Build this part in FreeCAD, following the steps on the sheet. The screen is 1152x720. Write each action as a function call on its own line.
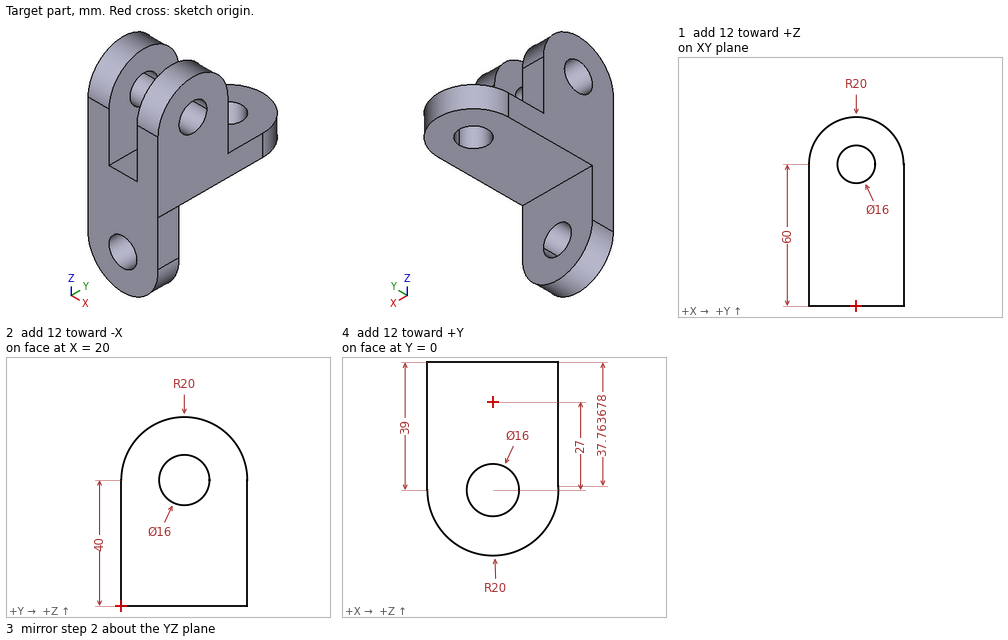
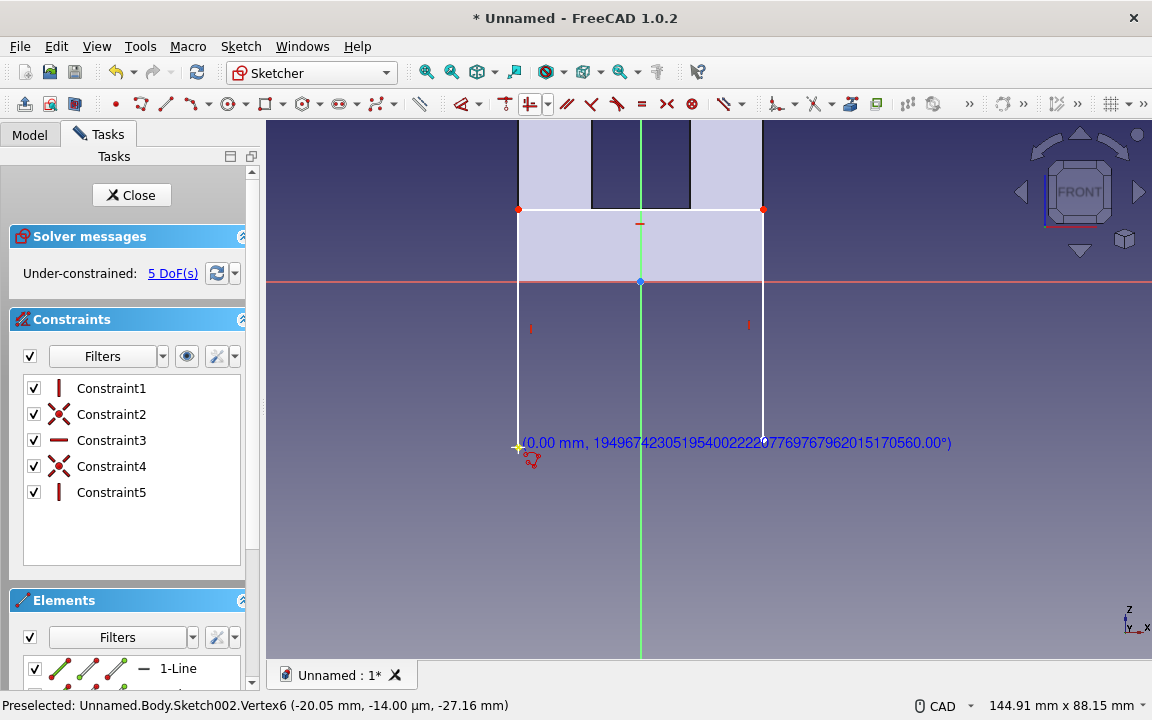
key(g)
key(3)
key(a)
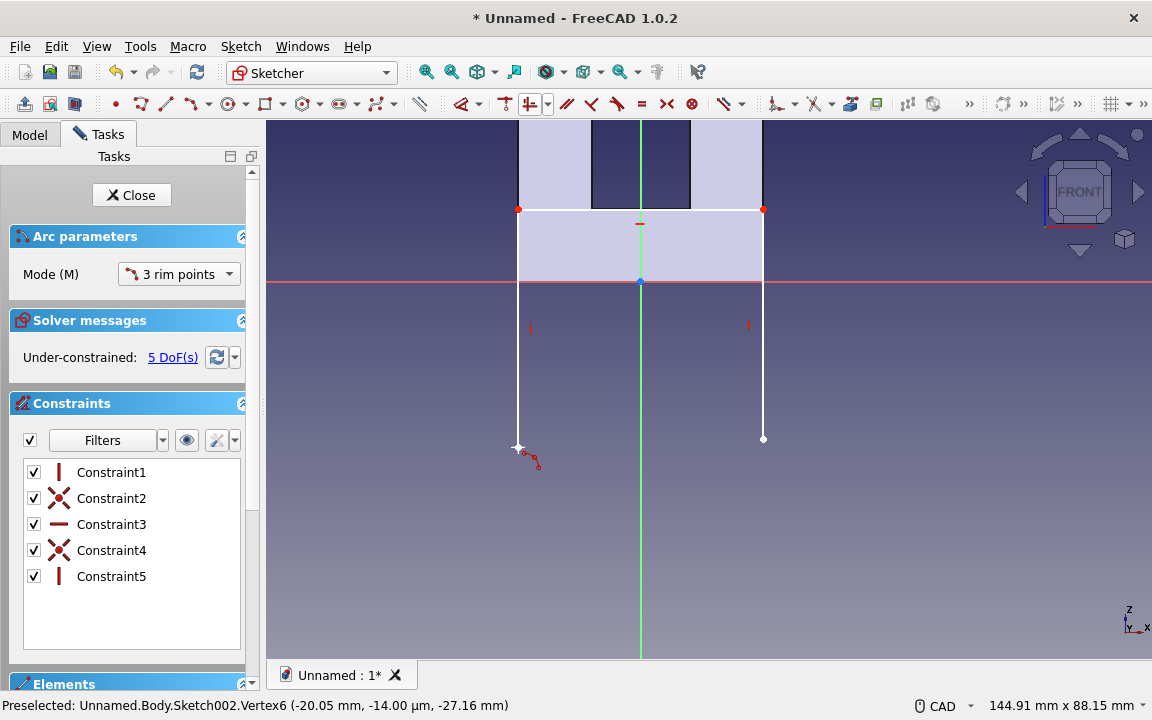
click(518, 448)
click(763, 440)
click(606, 564)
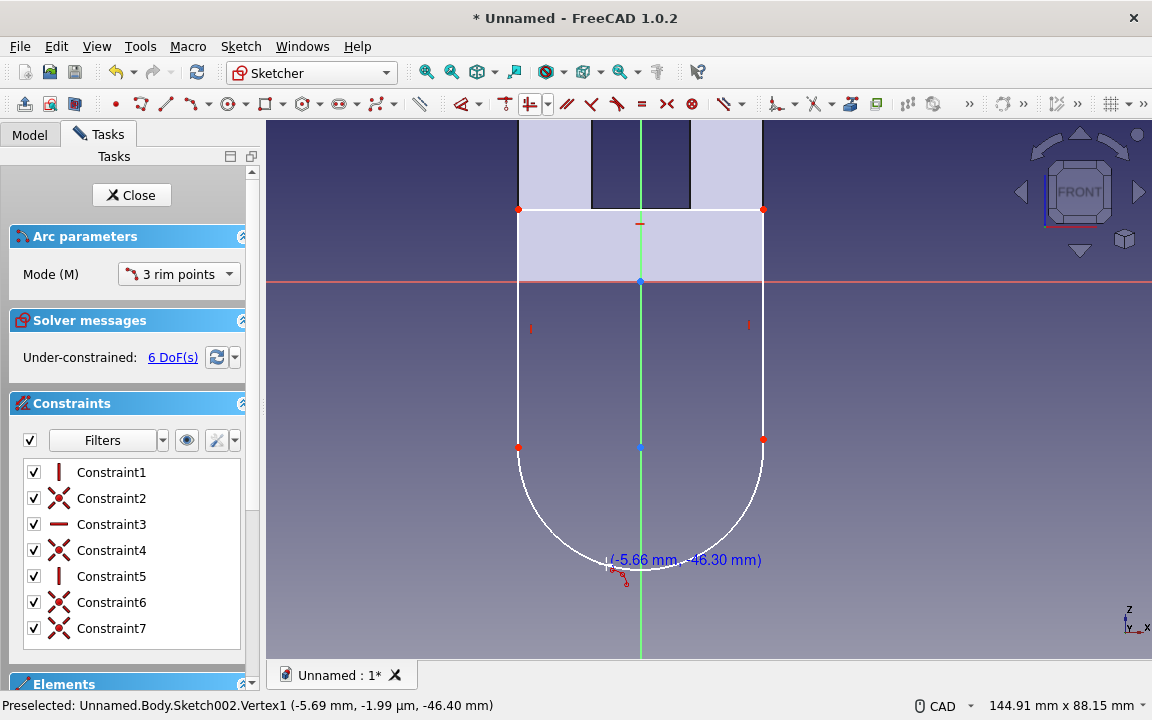
click(228, 104)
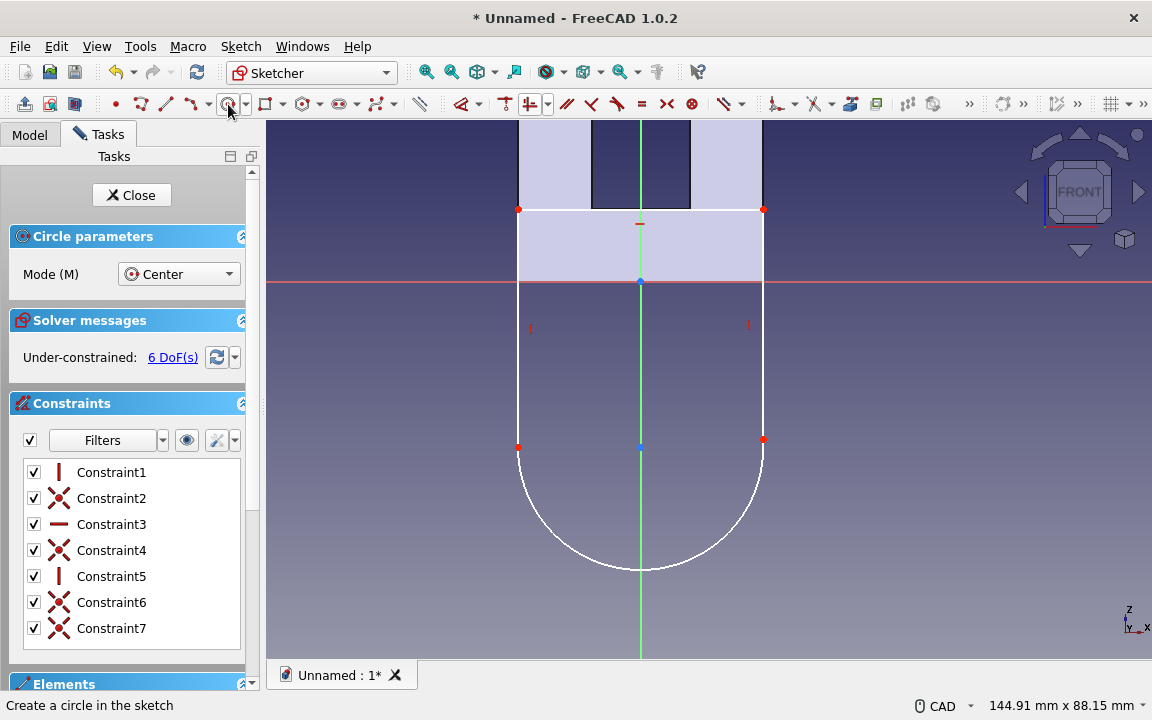
click(641, 447)
move(675, 412)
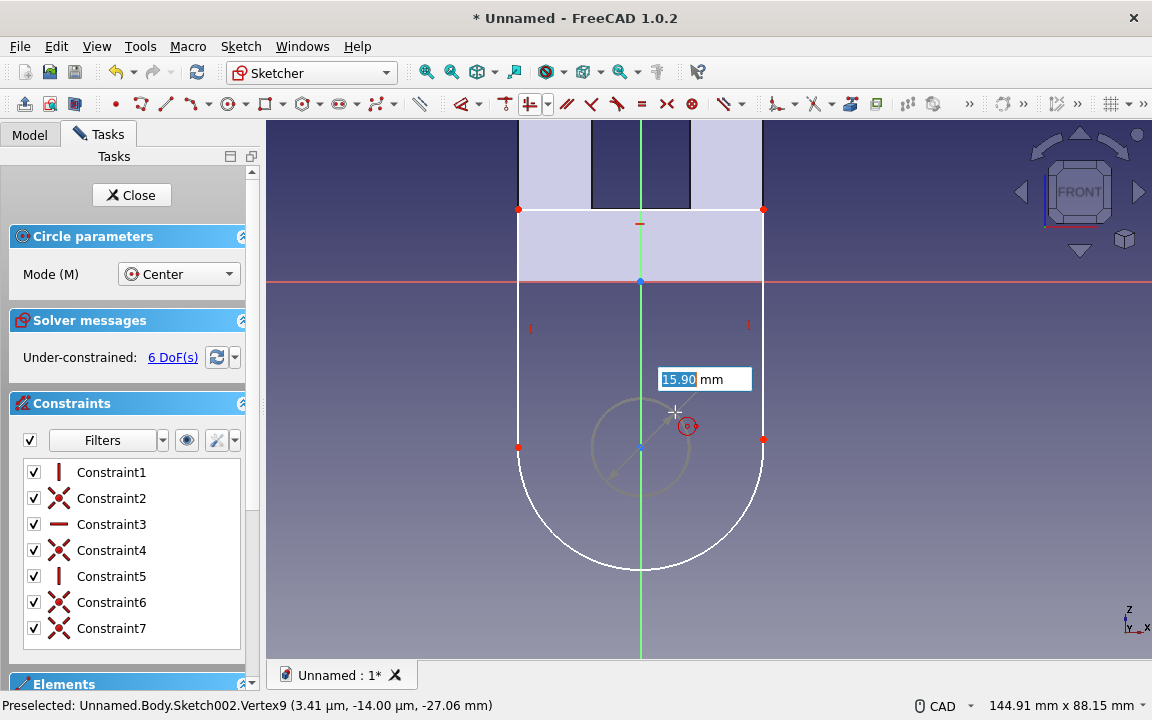
text(16)
key(Return)
key(Escape)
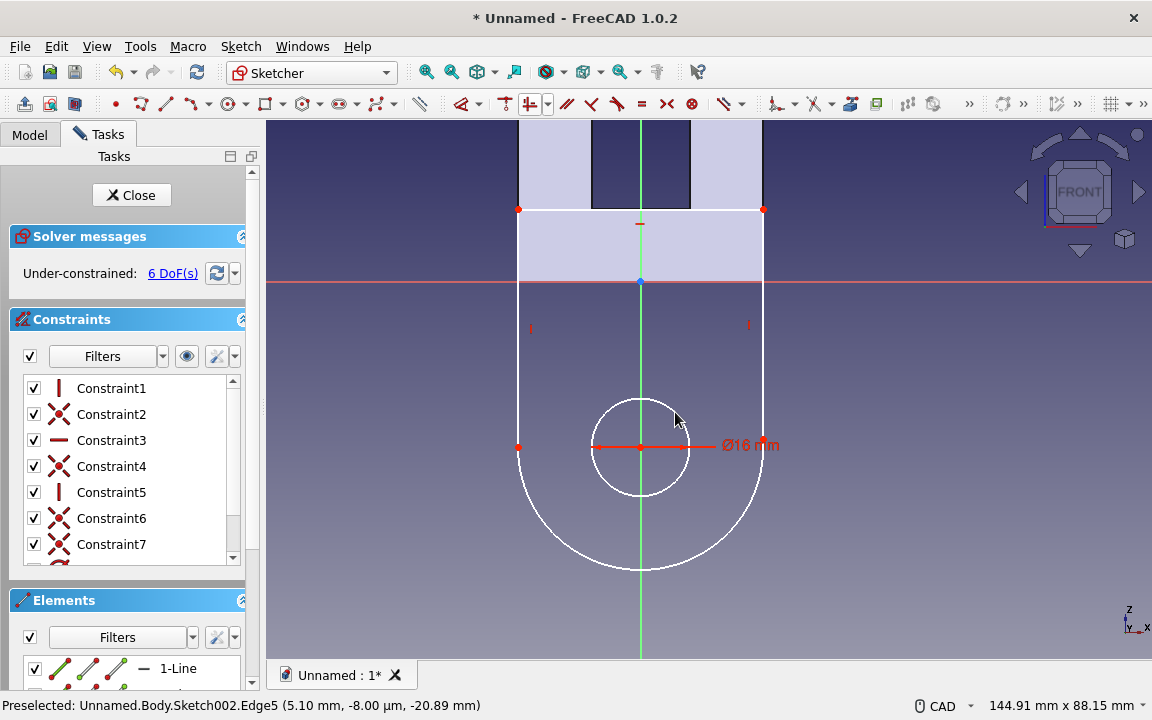
click(518, 281)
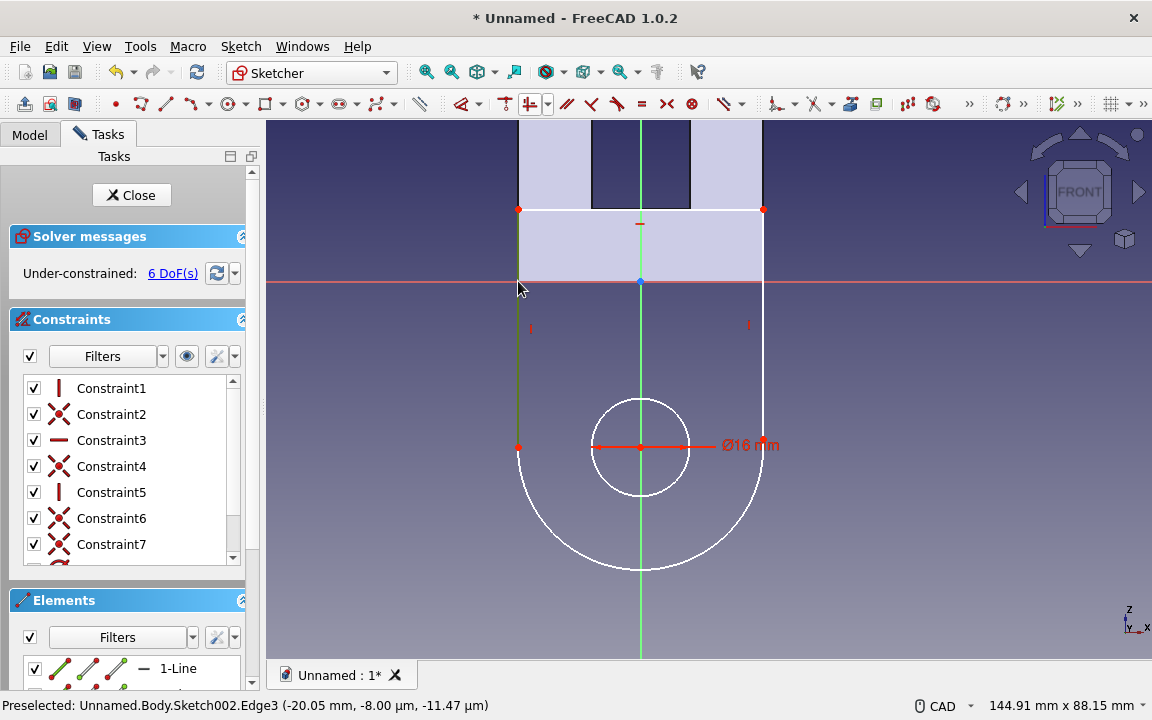
click(571, 548)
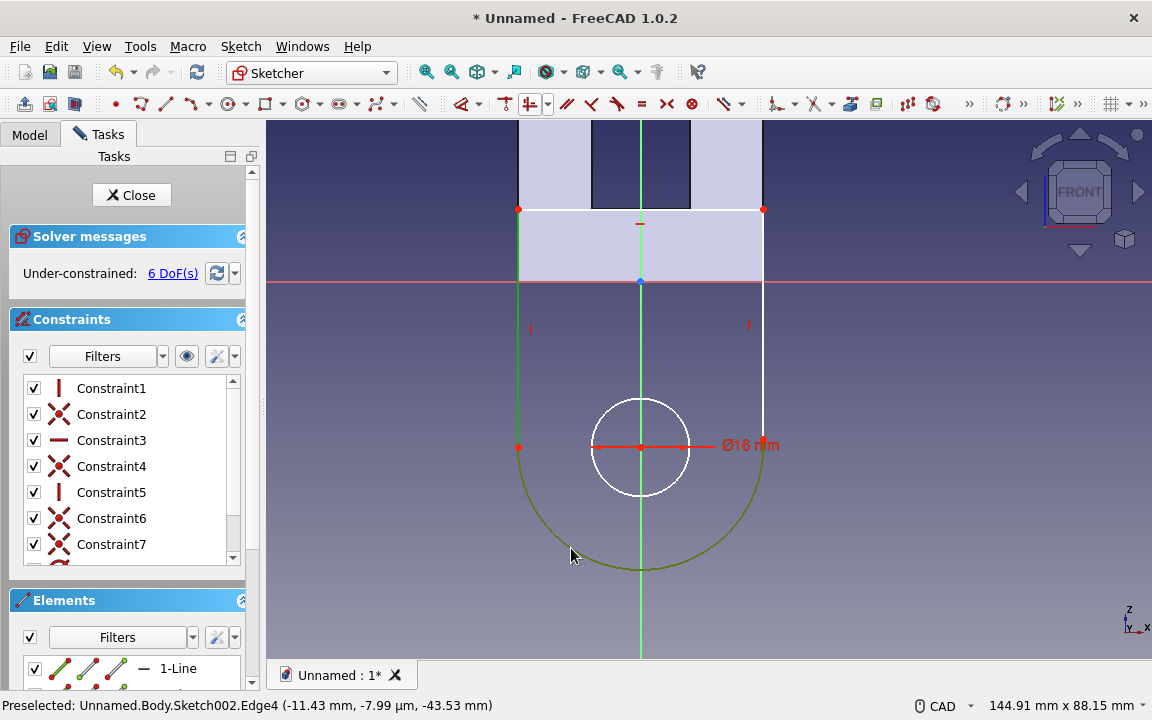
key(t)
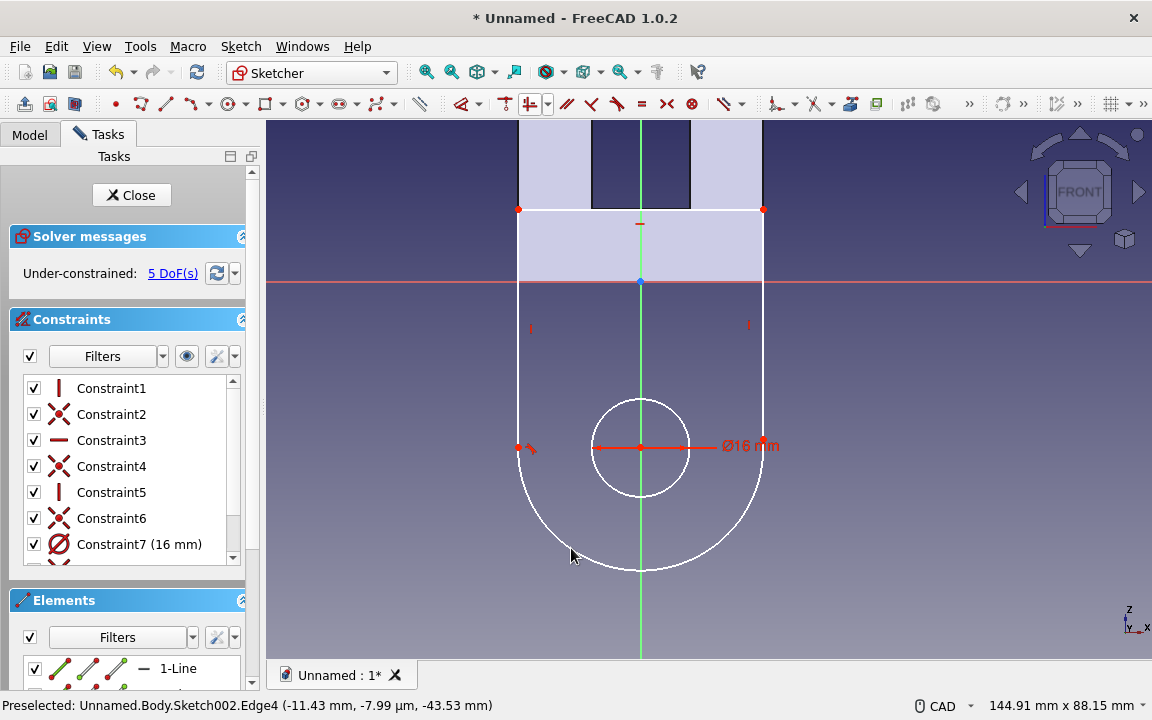
click(641, 448)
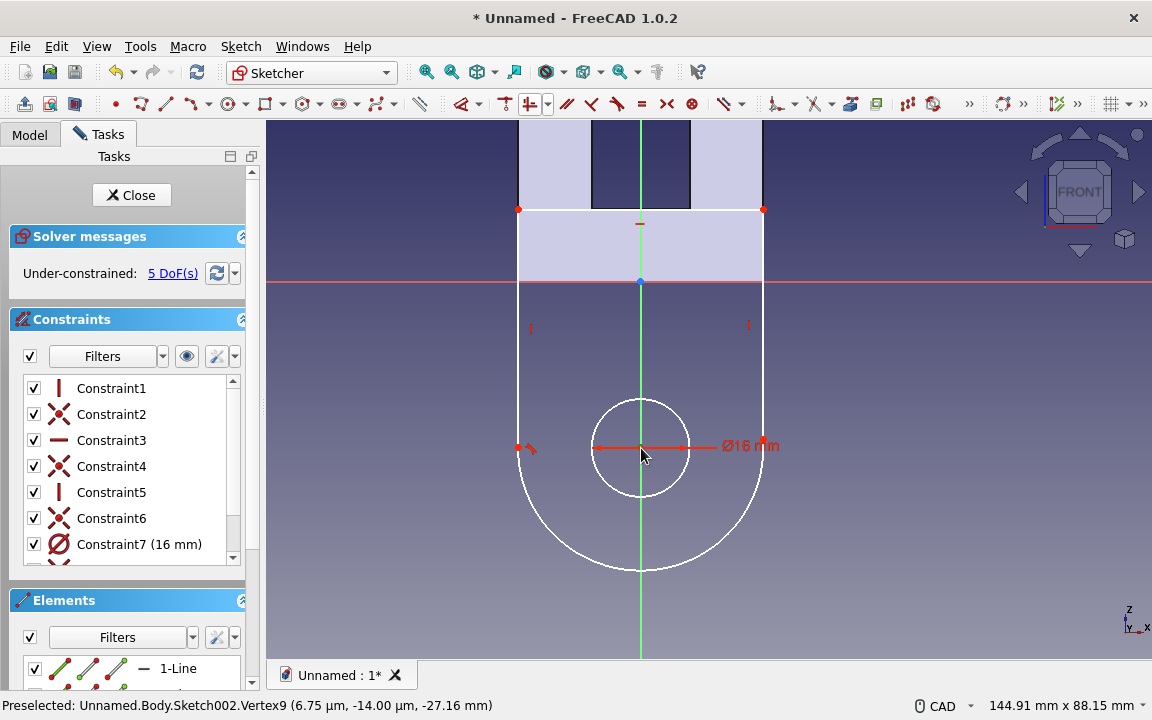
click(641, 528)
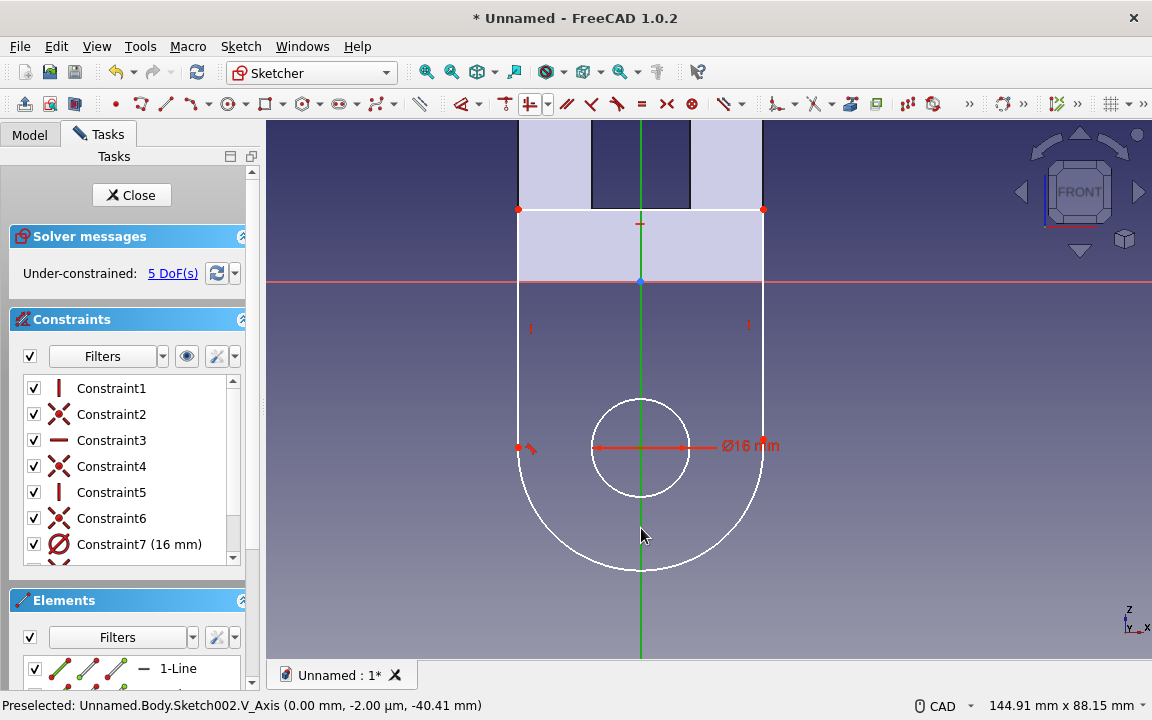
key(c)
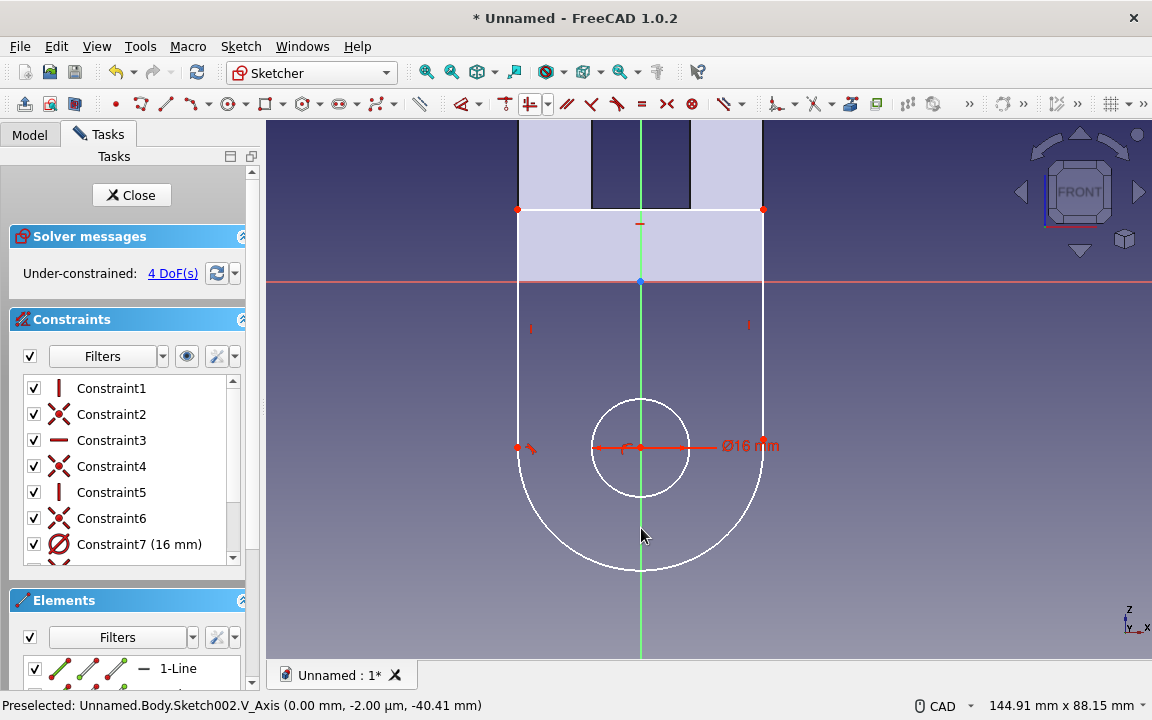
key(d)